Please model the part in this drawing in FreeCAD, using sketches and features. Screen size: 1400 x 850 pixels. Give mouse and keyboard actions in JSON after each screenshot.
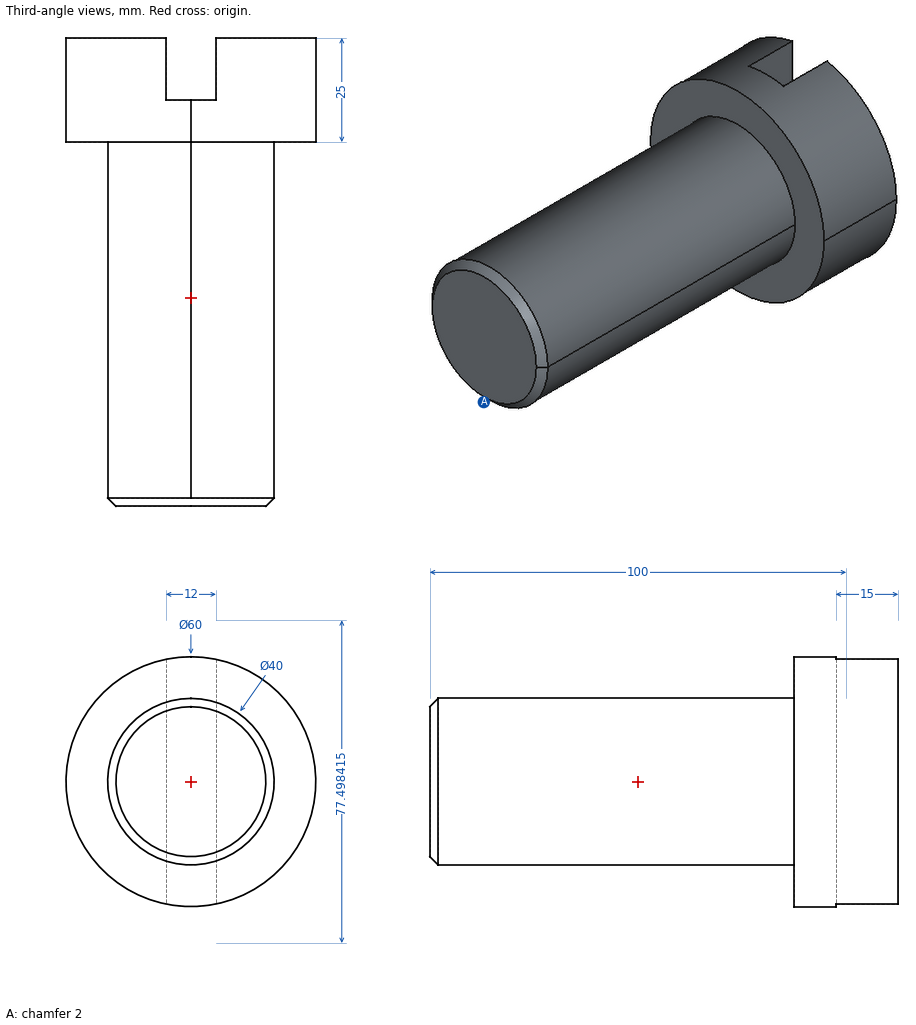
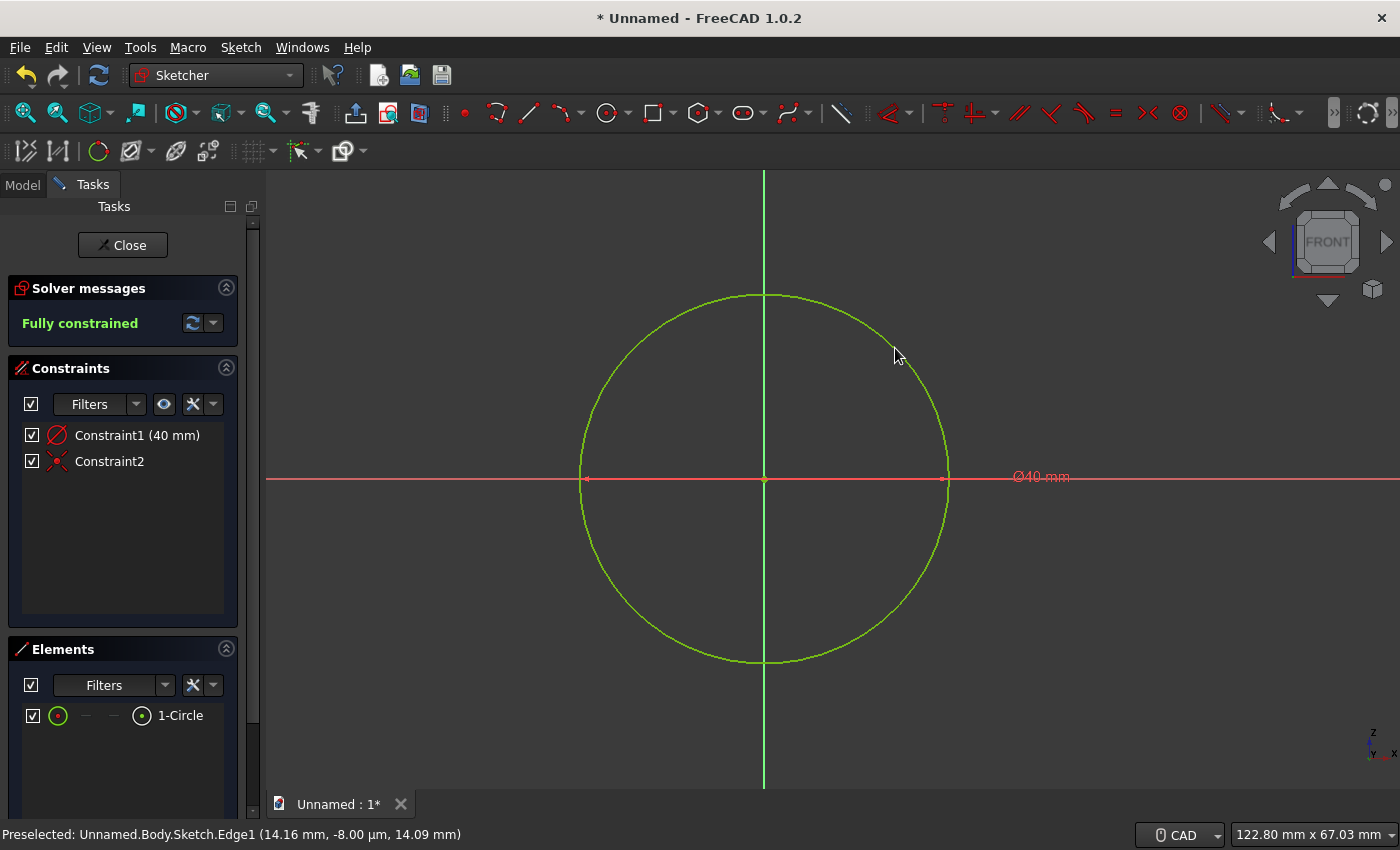
{"action": "left_click", "coordinate": [123, 245]}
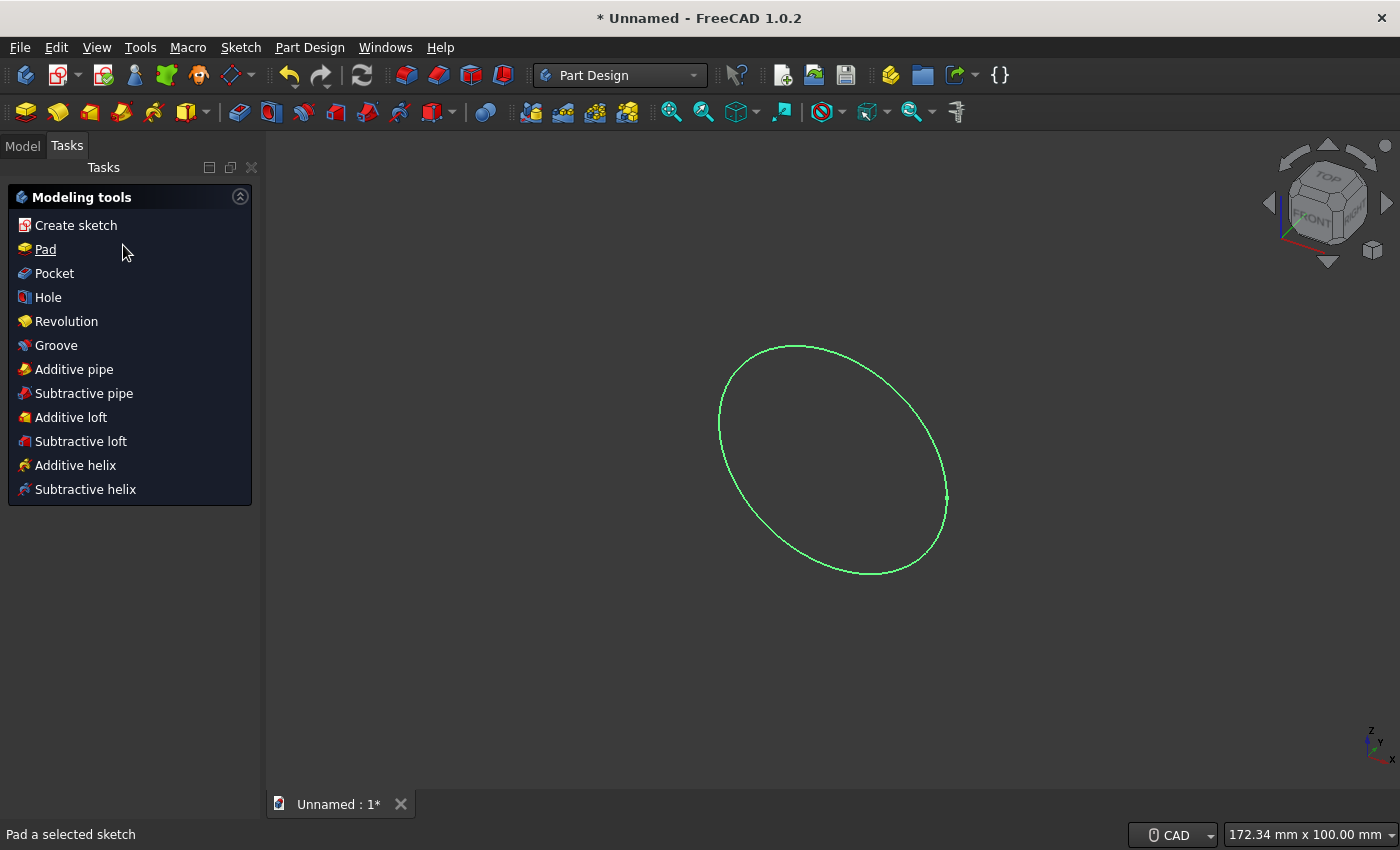
{"action": "left_click", "coordinate": [26, 112]}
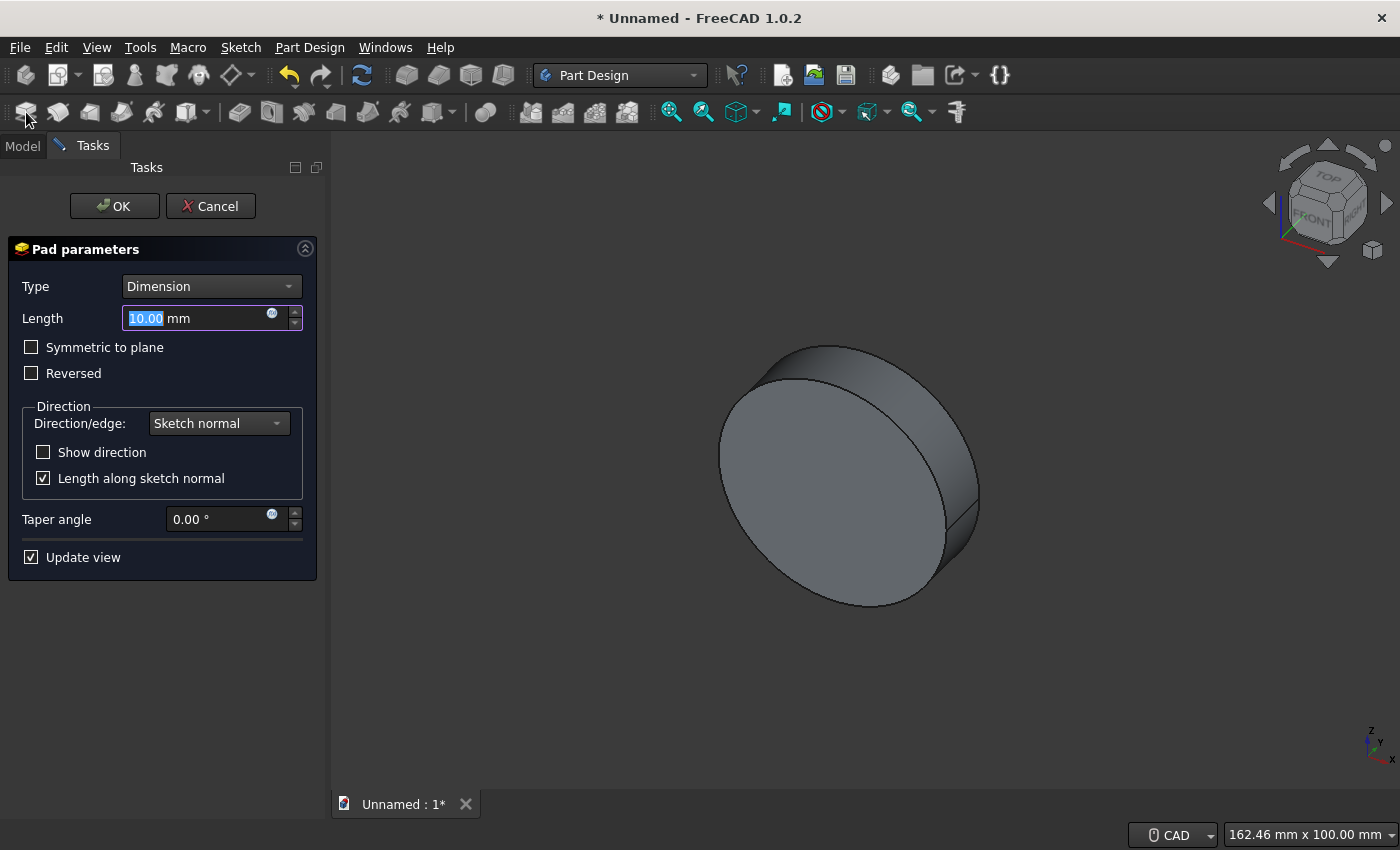
{"action": "type", "text": "100"}
{"action": "key", "text": "Tab"}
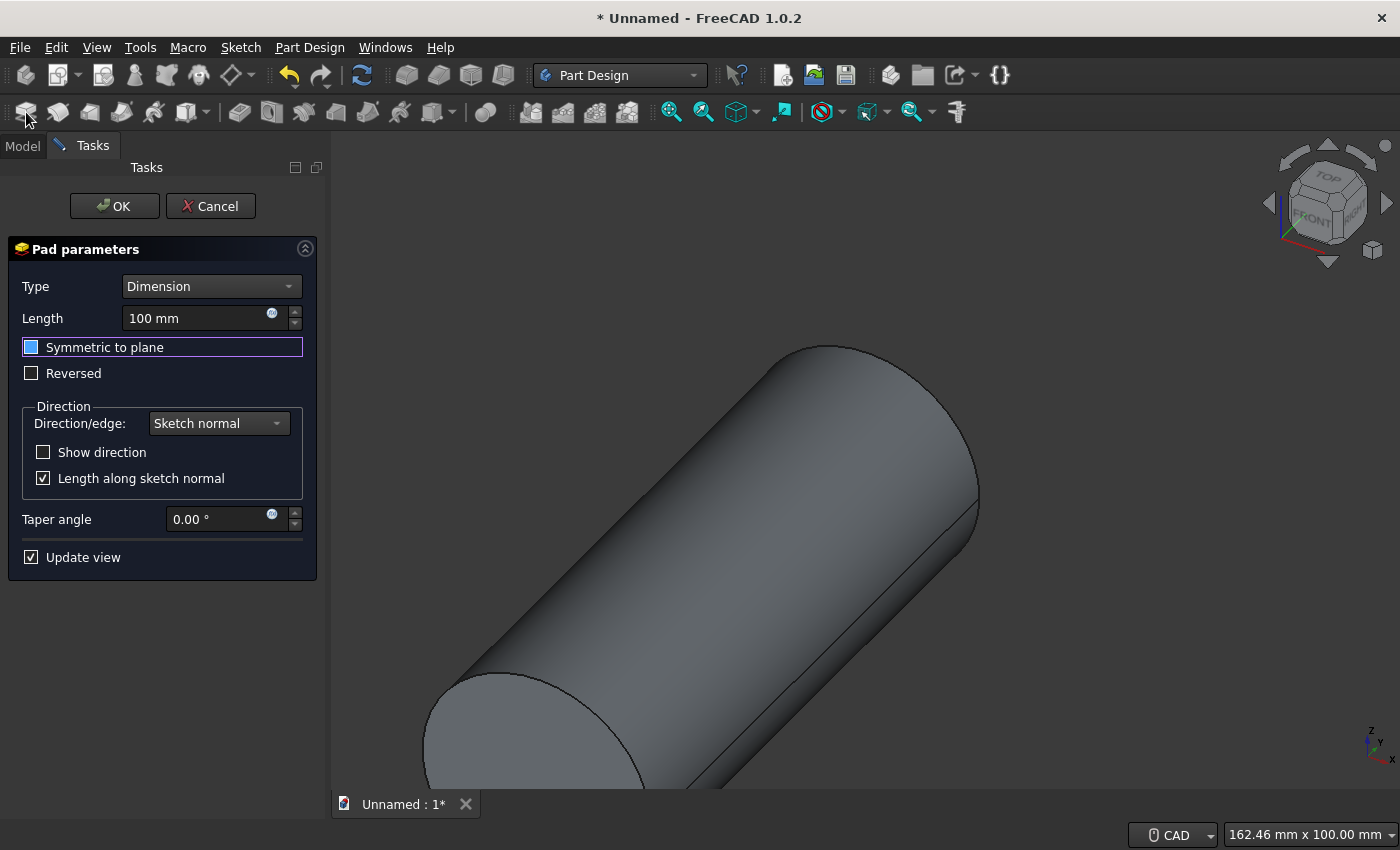
{"action": "left_click", "coordinate": [30, 347]}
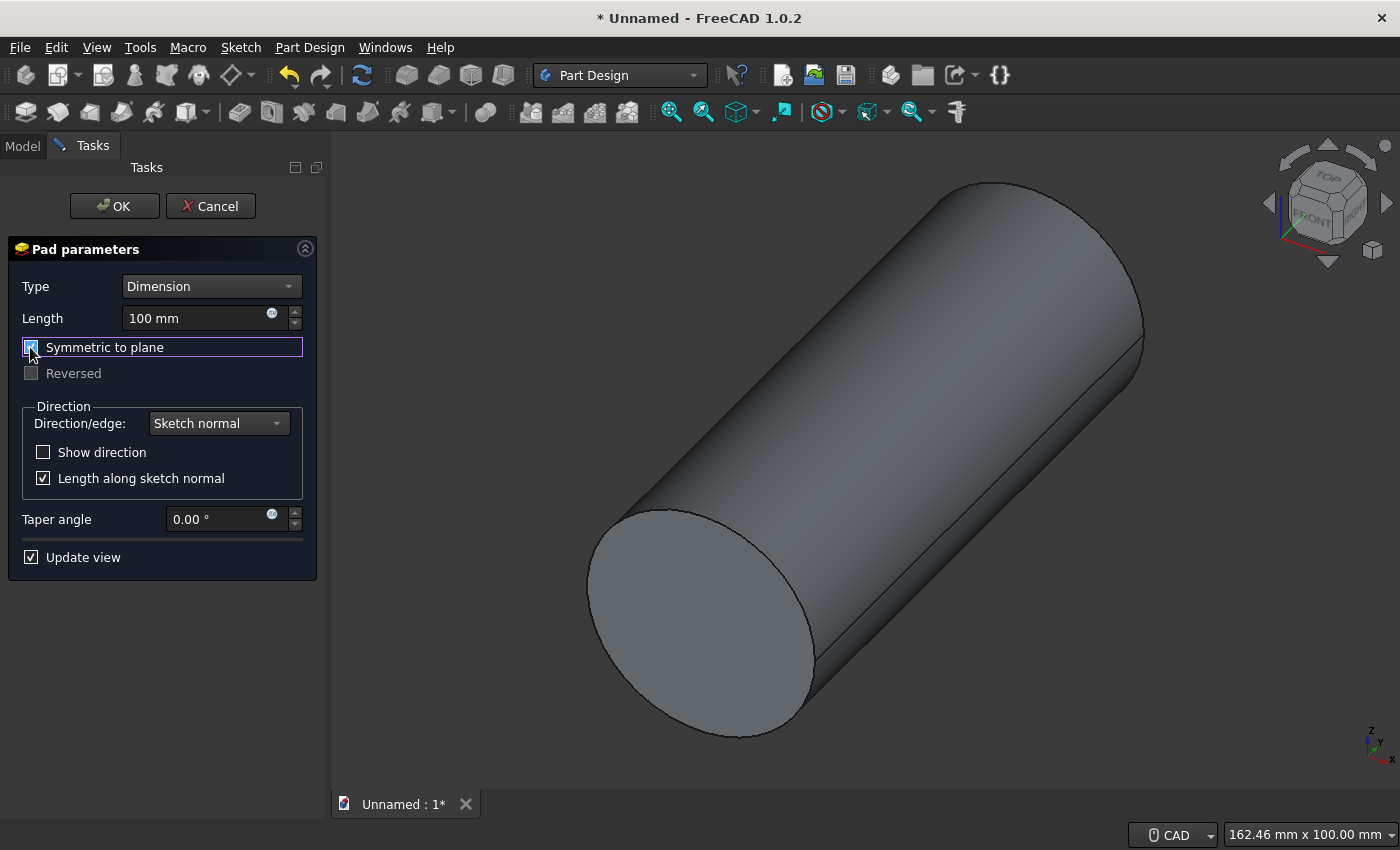
{"action": "left_click", "coordinate": [115, 206]}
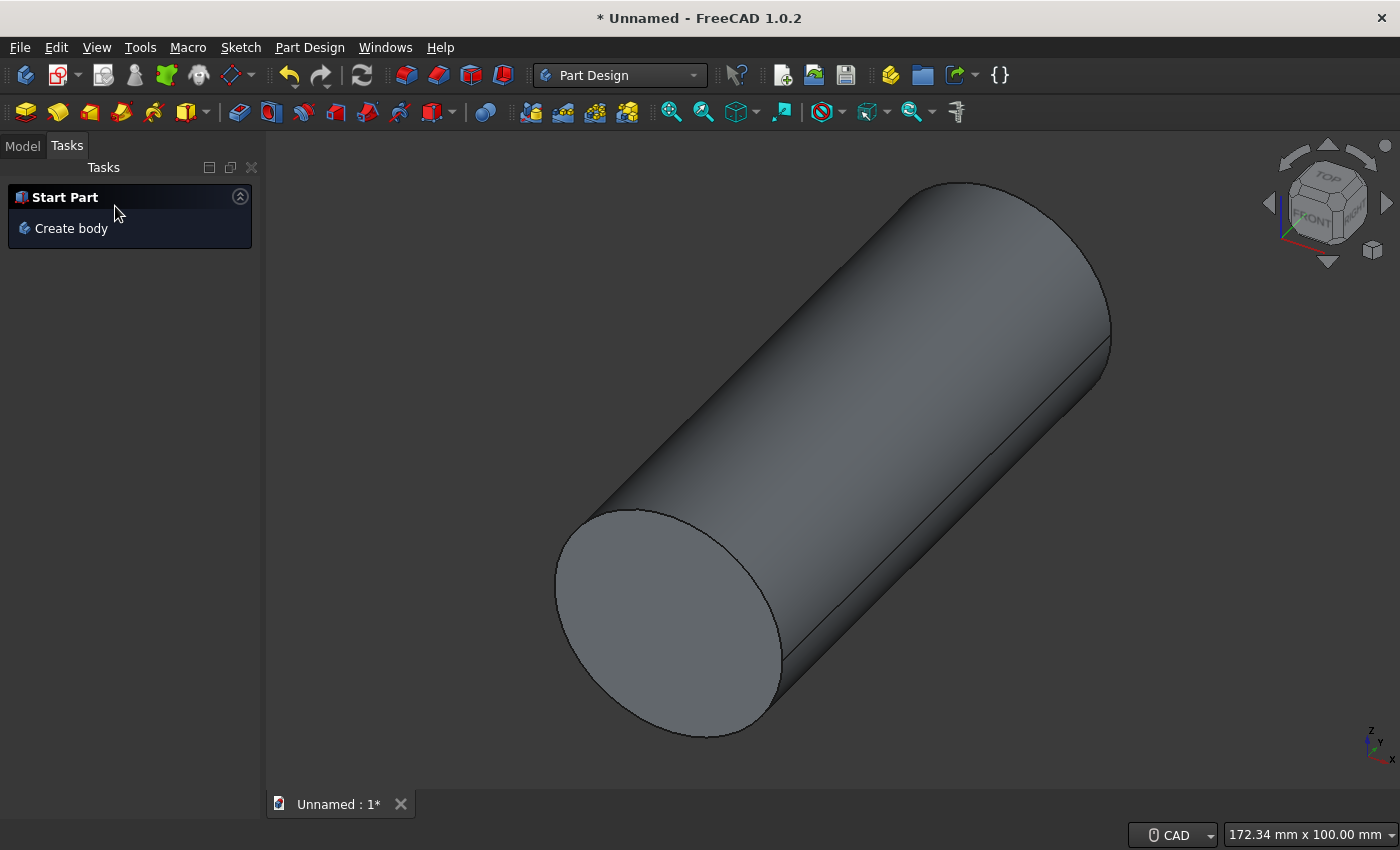
{"action": "key", "text": "4"}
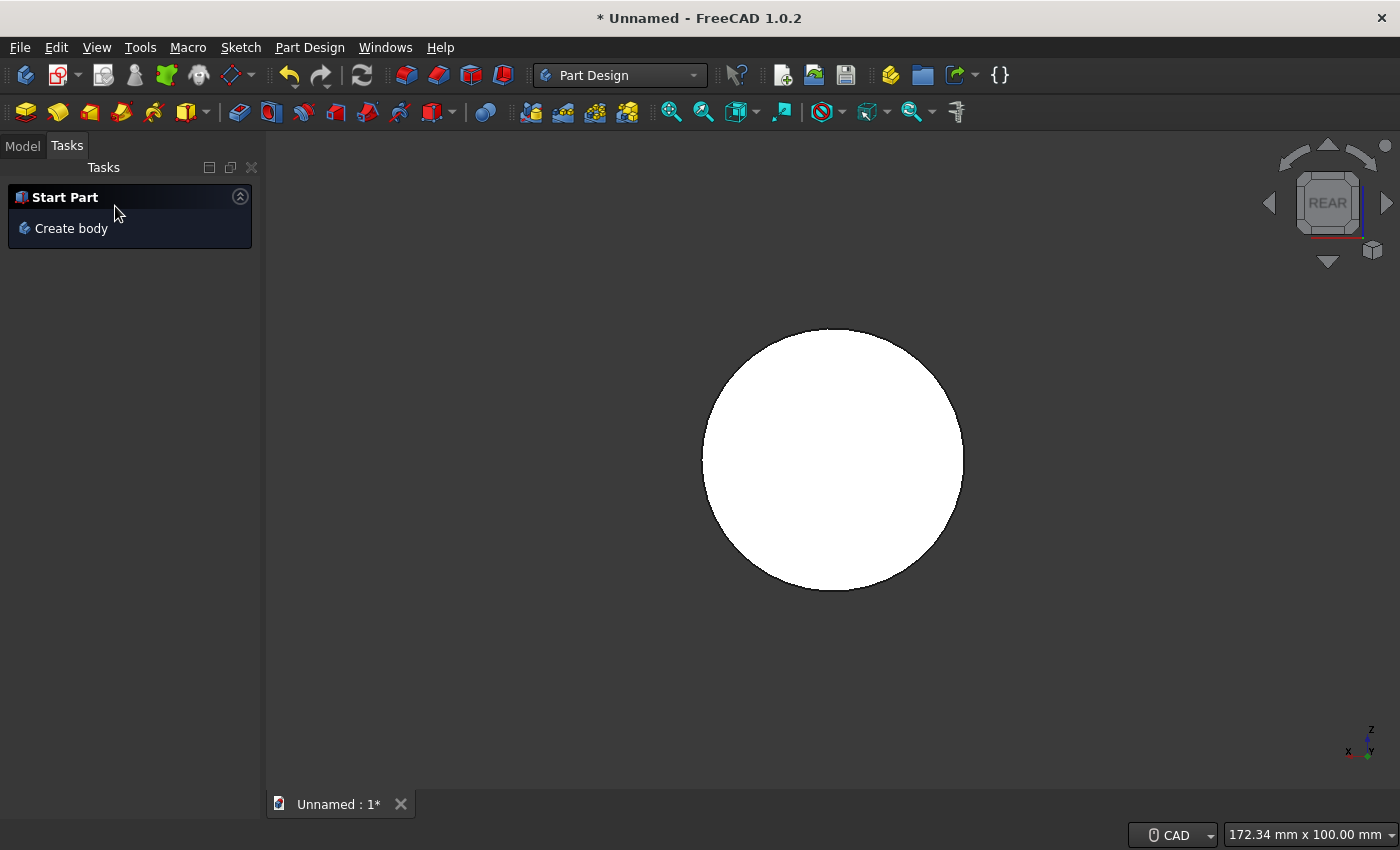
{"action": "left_click", "coordinate": [672, 112]}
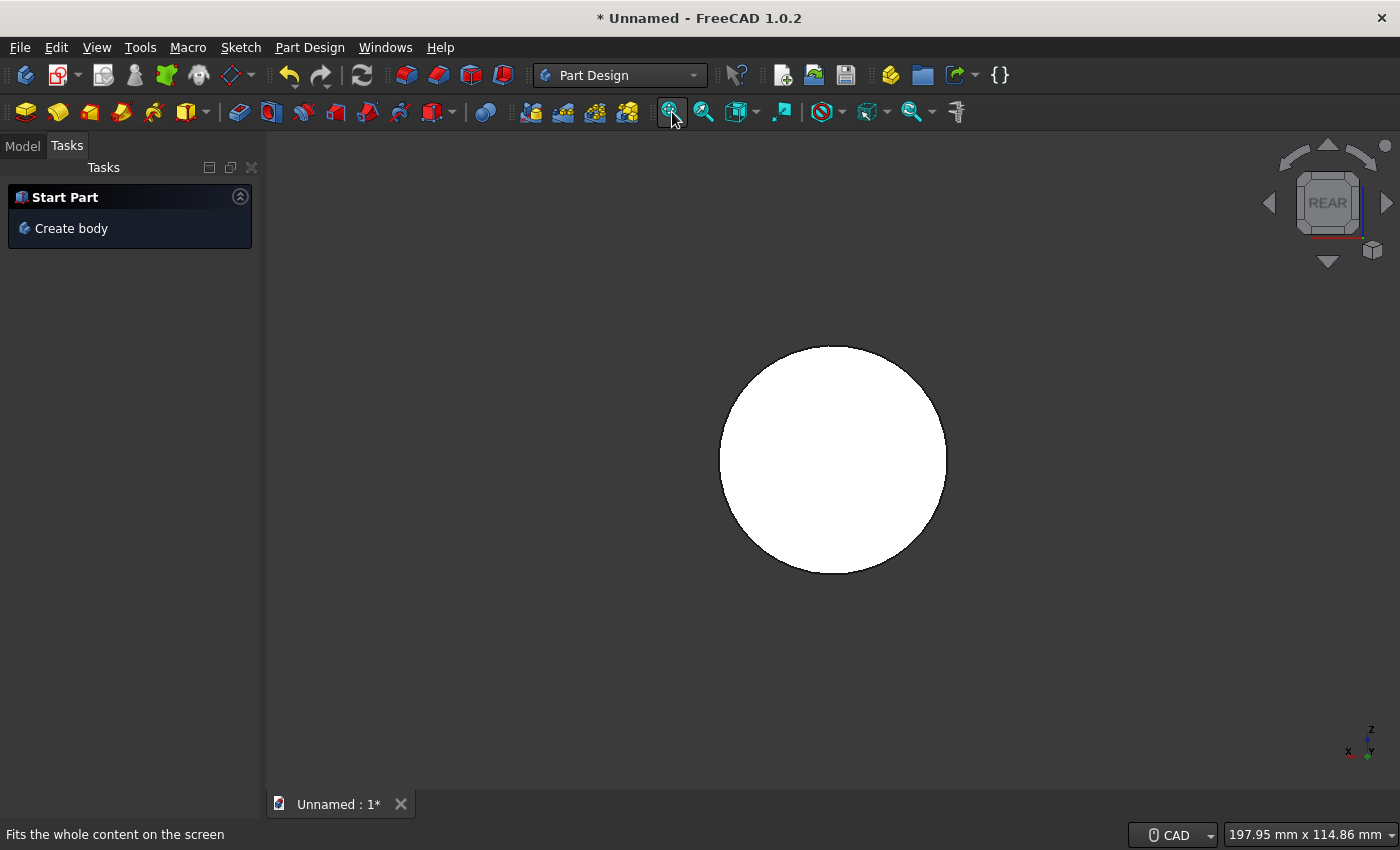
{"action": "left_click", "coordinate": [833, 459]}